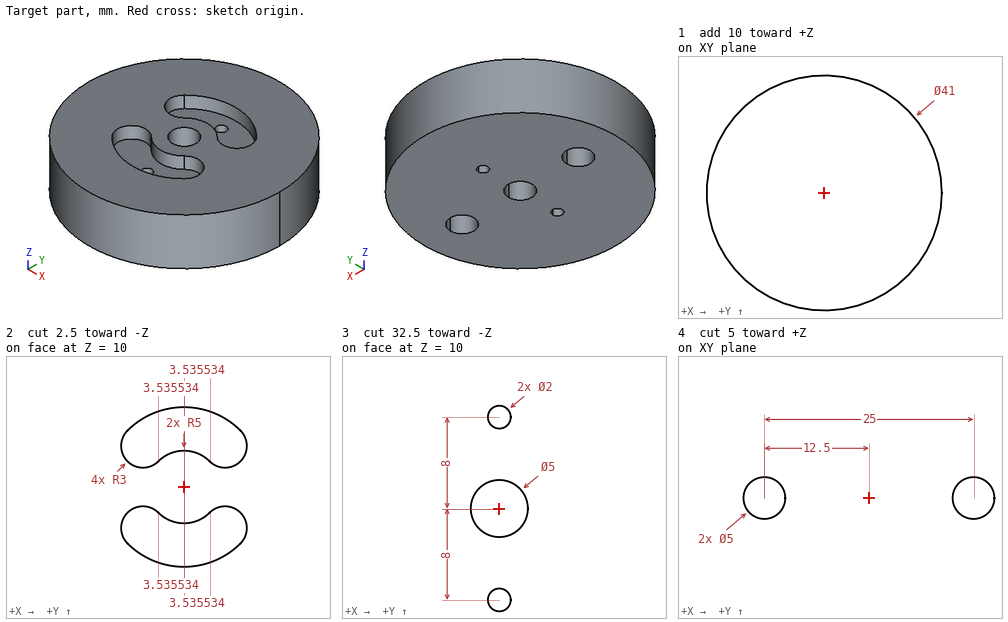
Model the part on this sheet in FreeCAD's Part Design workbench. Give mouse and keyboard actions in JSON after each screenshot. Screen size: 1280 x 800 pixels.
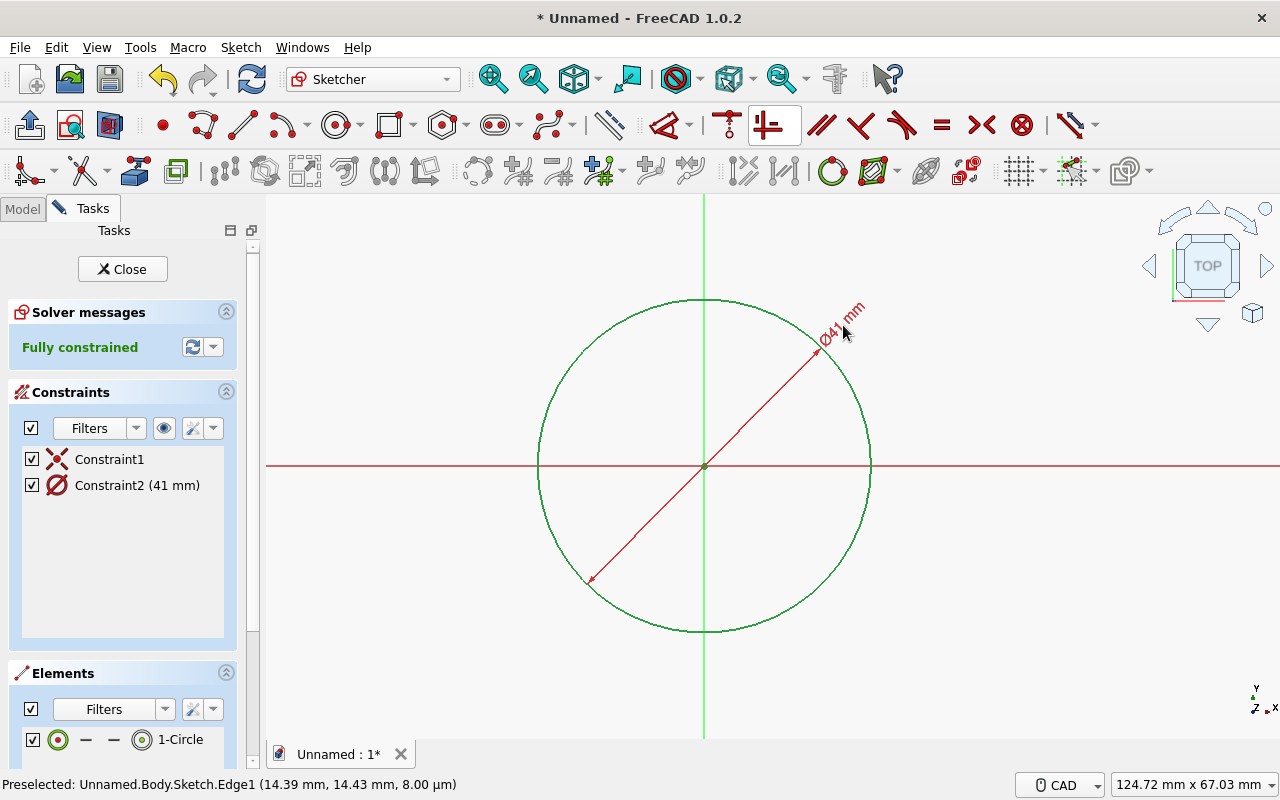
{"action": "left_click", "coordinate": [123, 269]}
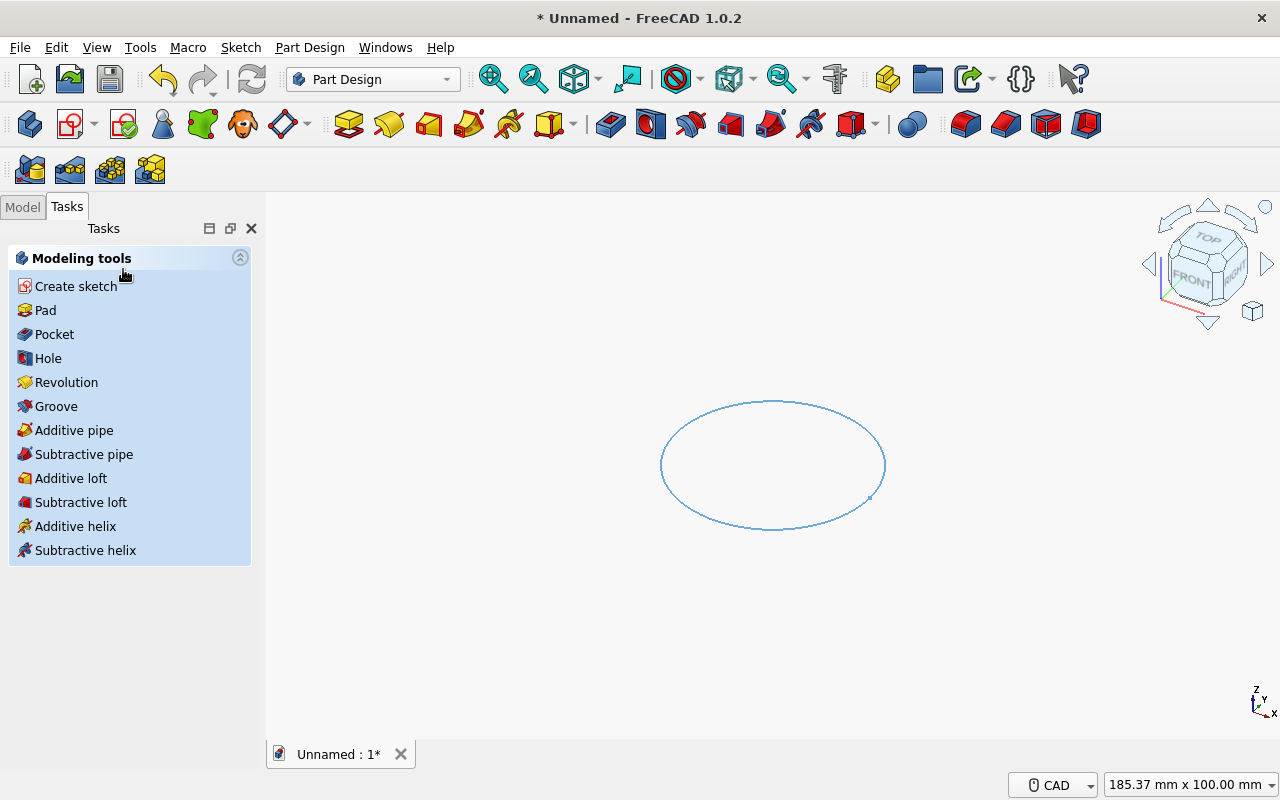
{"action": "left_click", "coordinate": [350, 124]}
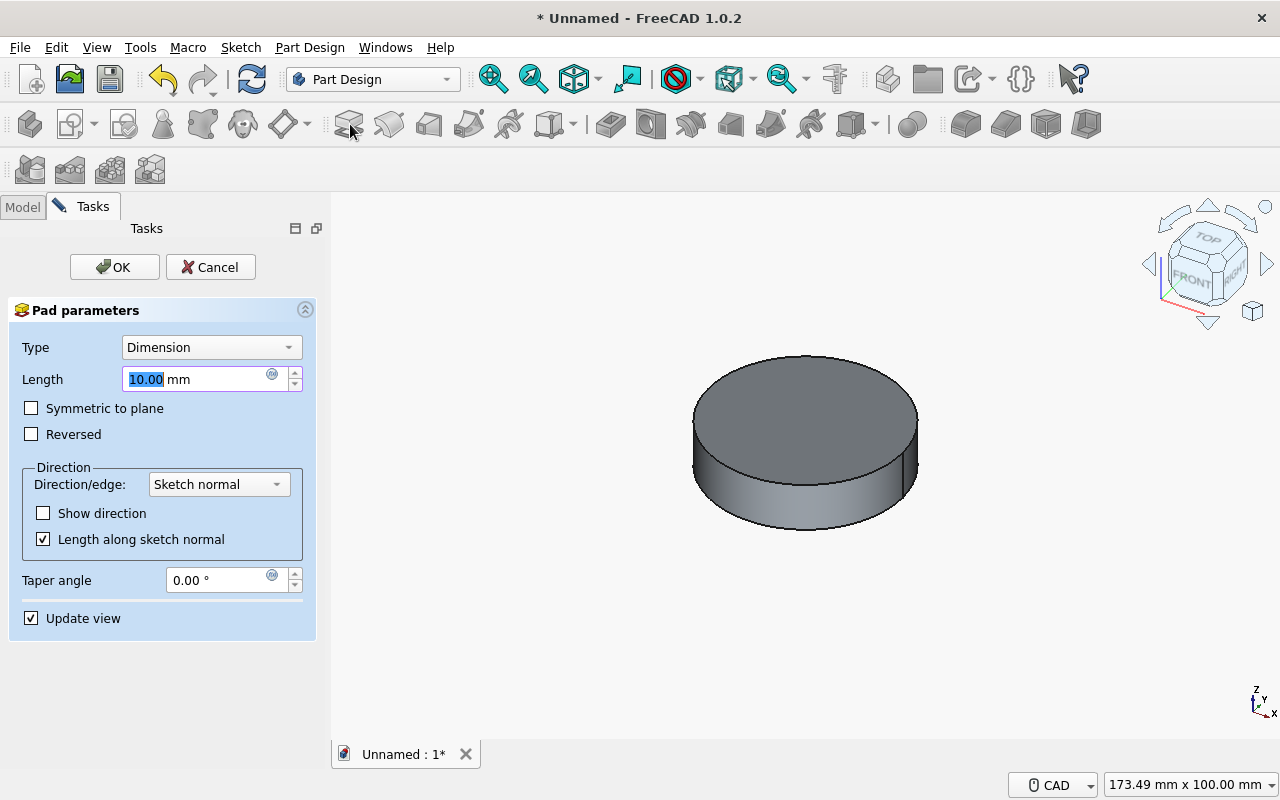
{"action": "type", "text": "10"}
{"action": "key", "text": "Tab"}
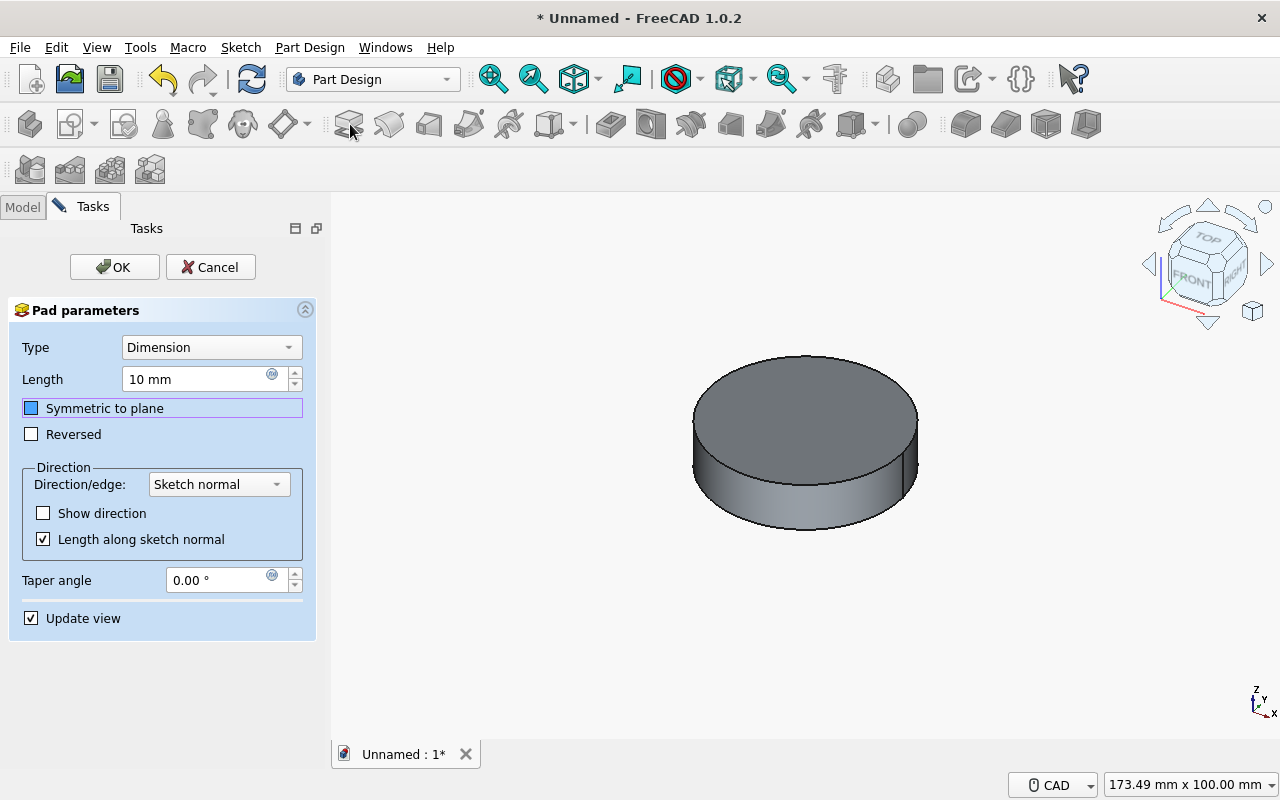
{"action": "left_click", "coordinate": [115, 267]}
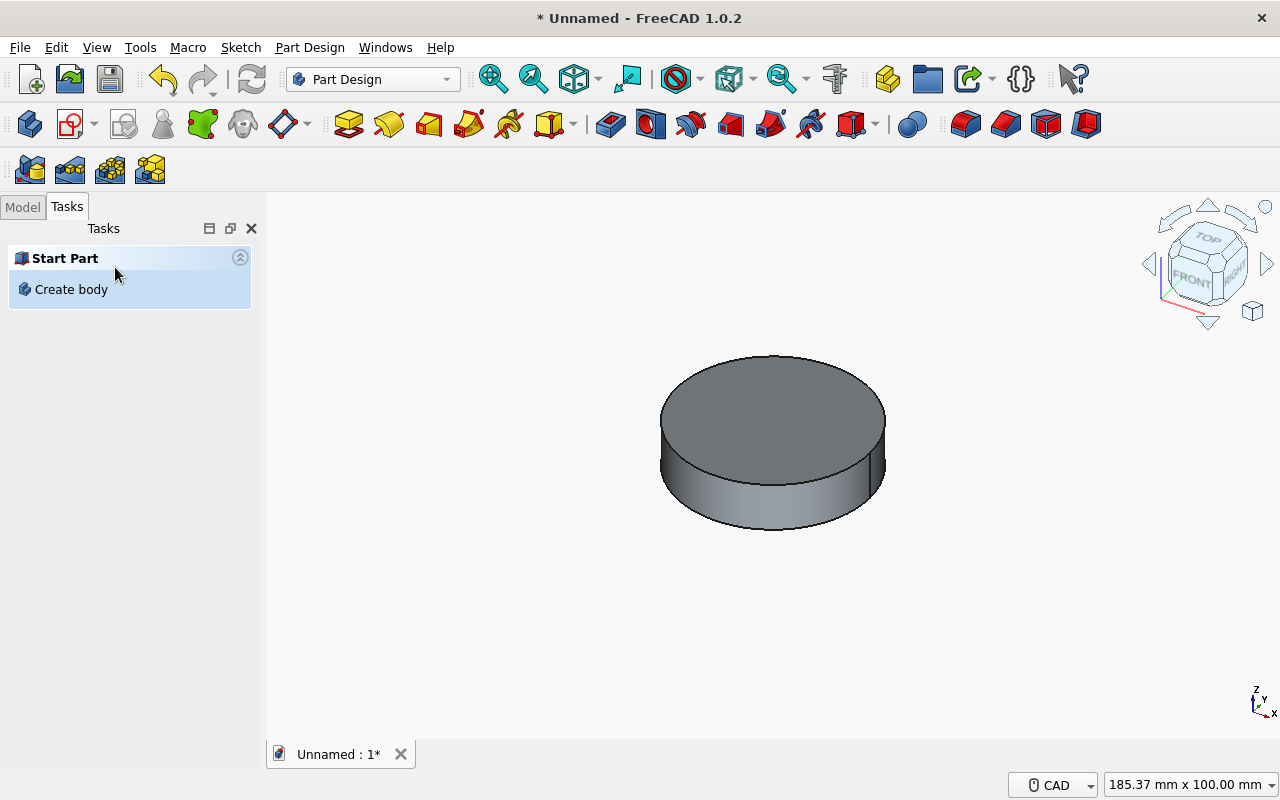
{"action": "left_click", "coordinate": [494, 80]}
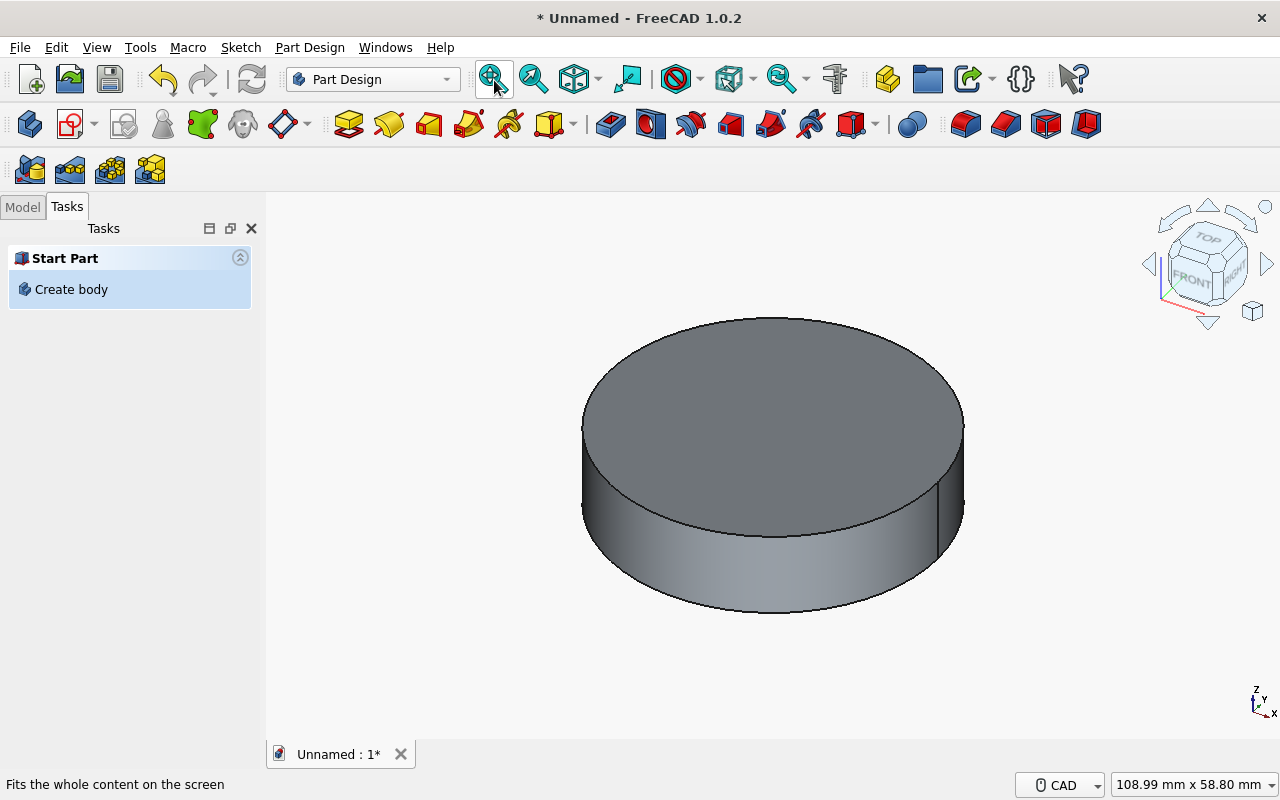
{"action": "left_click", "coordinate": [773, 426]}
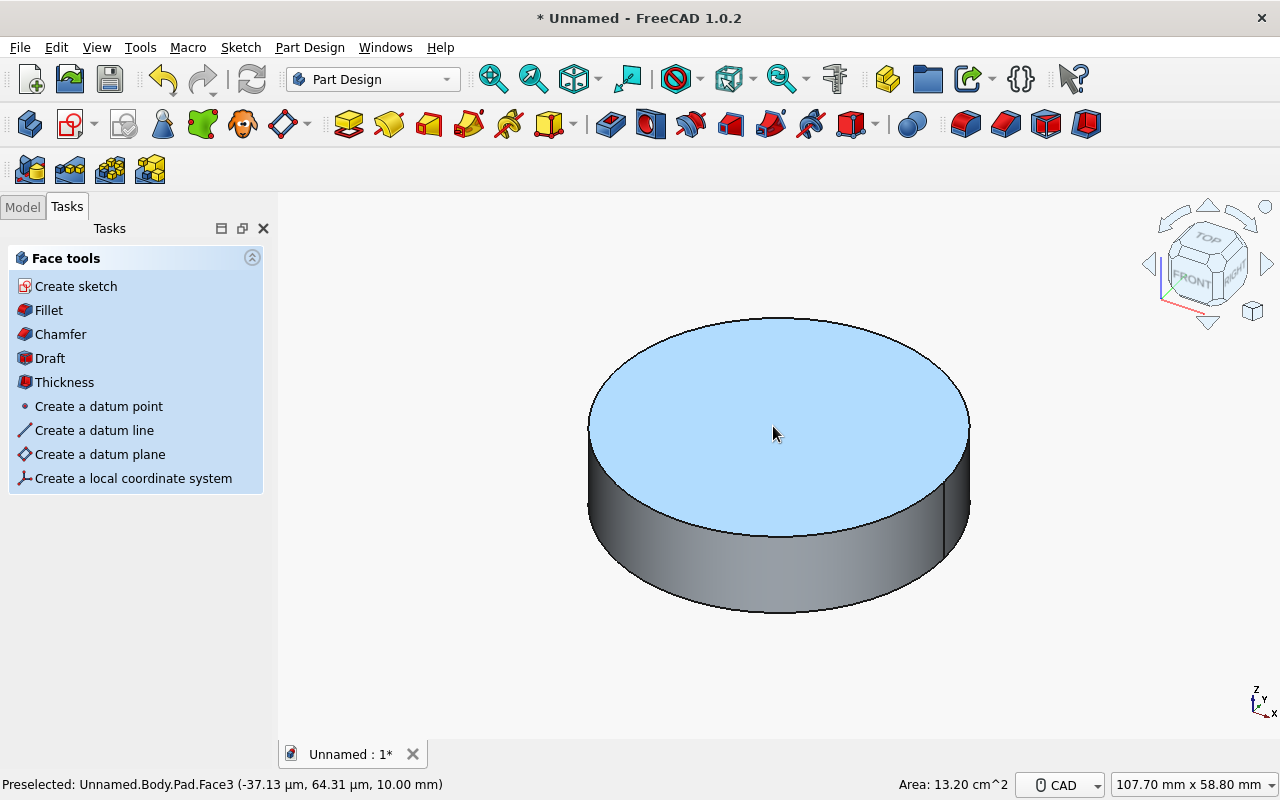
{"action": "left_click", "coordinate": [70, 124]}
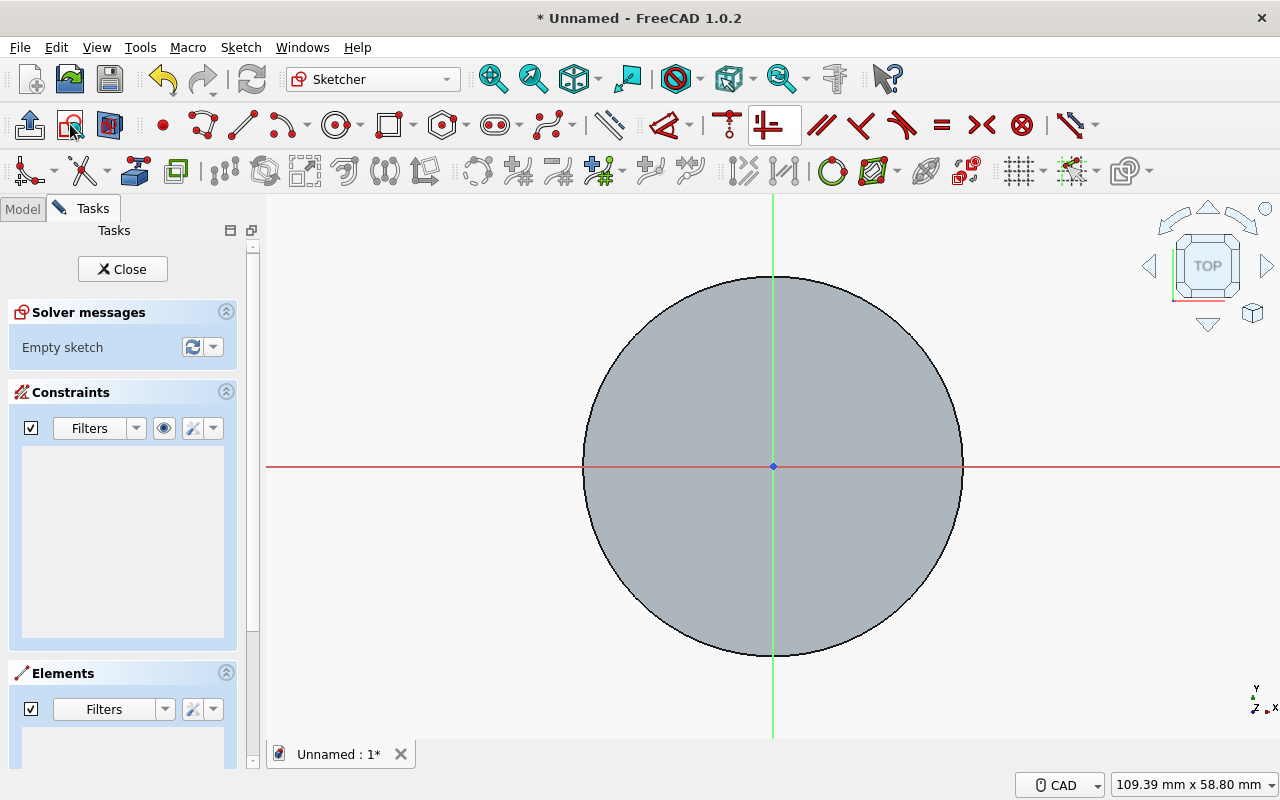
{"action": "scroll", "coordinate": [856, 466], "scroll_direction": "up", "scroll_amount": 3}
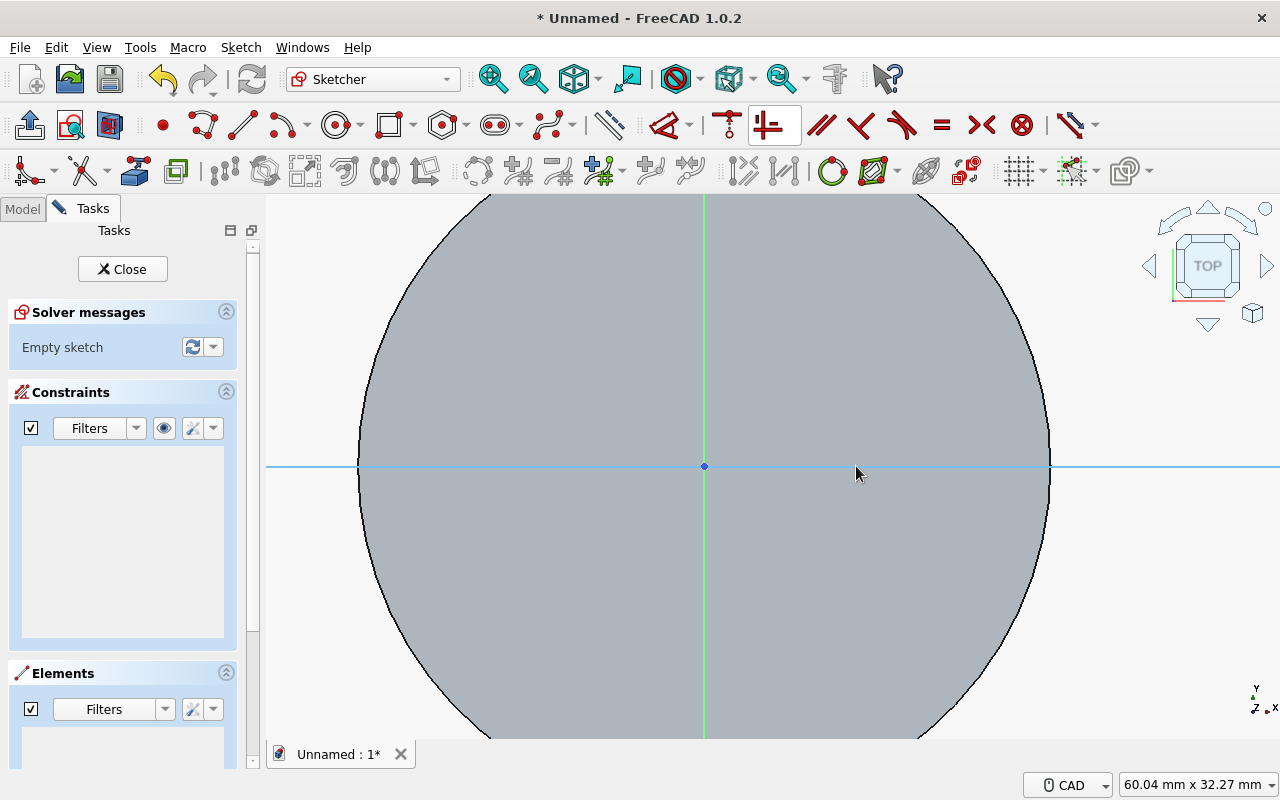
{"action": "key", "text": "g 3 a"}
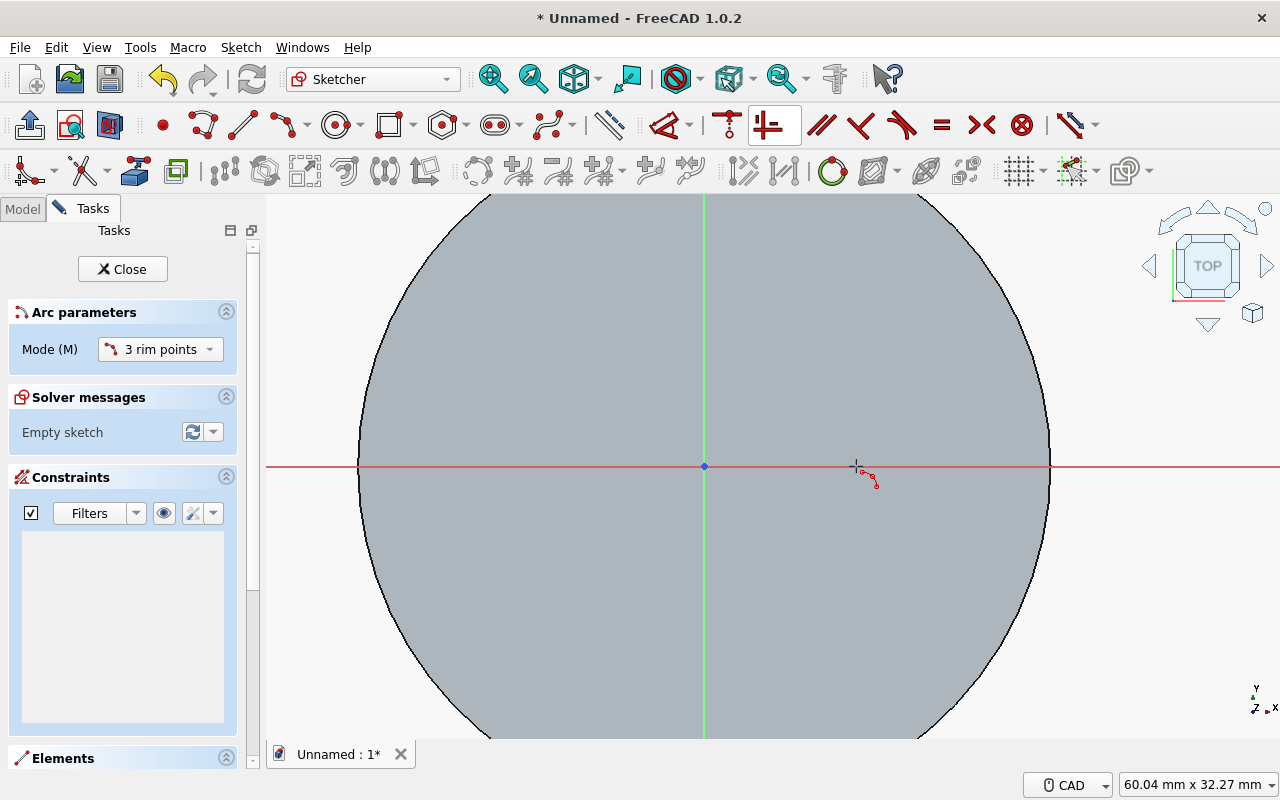
{"action": "left_click", "coordinate": [645, 407]}
{"action": "left_click", "coordinate": [764, 407]}
{"action": "left_click", "coordinate": [730, 386]}